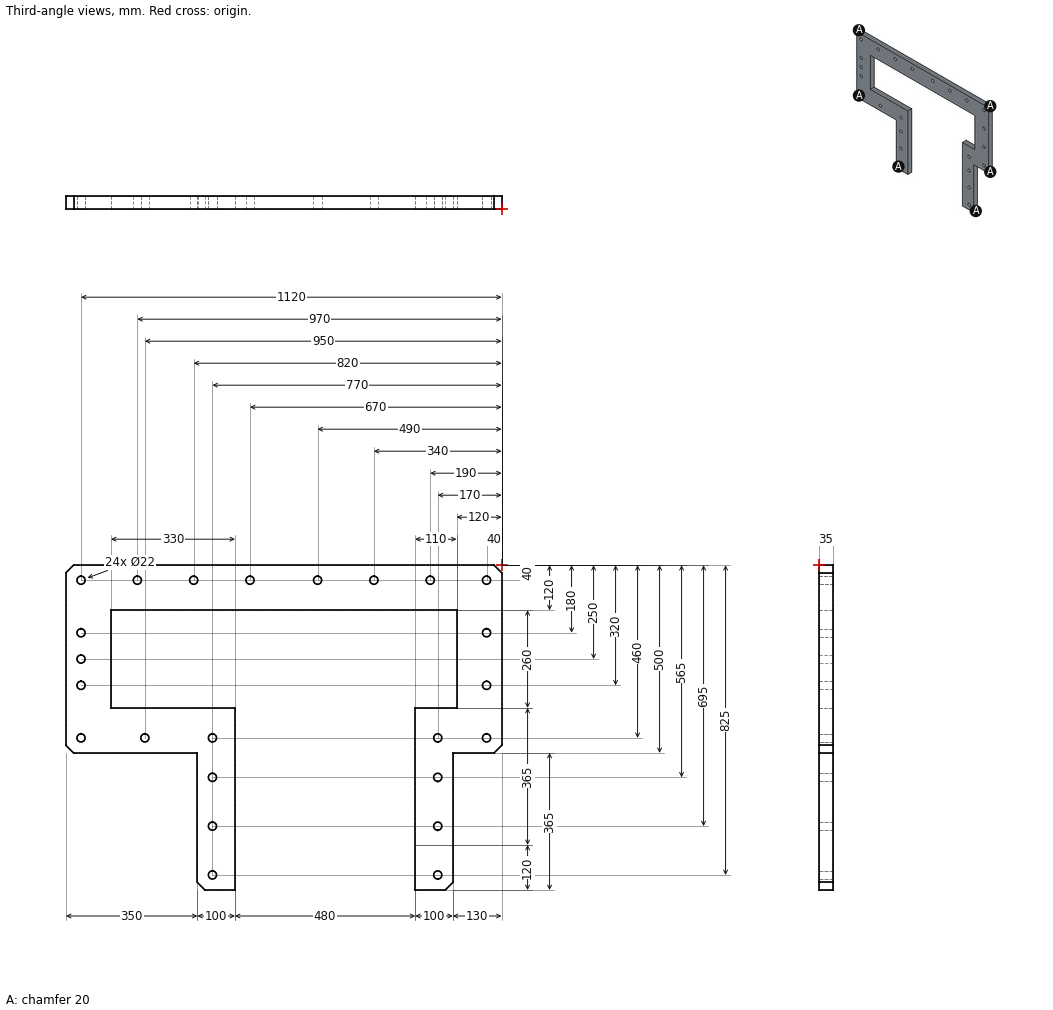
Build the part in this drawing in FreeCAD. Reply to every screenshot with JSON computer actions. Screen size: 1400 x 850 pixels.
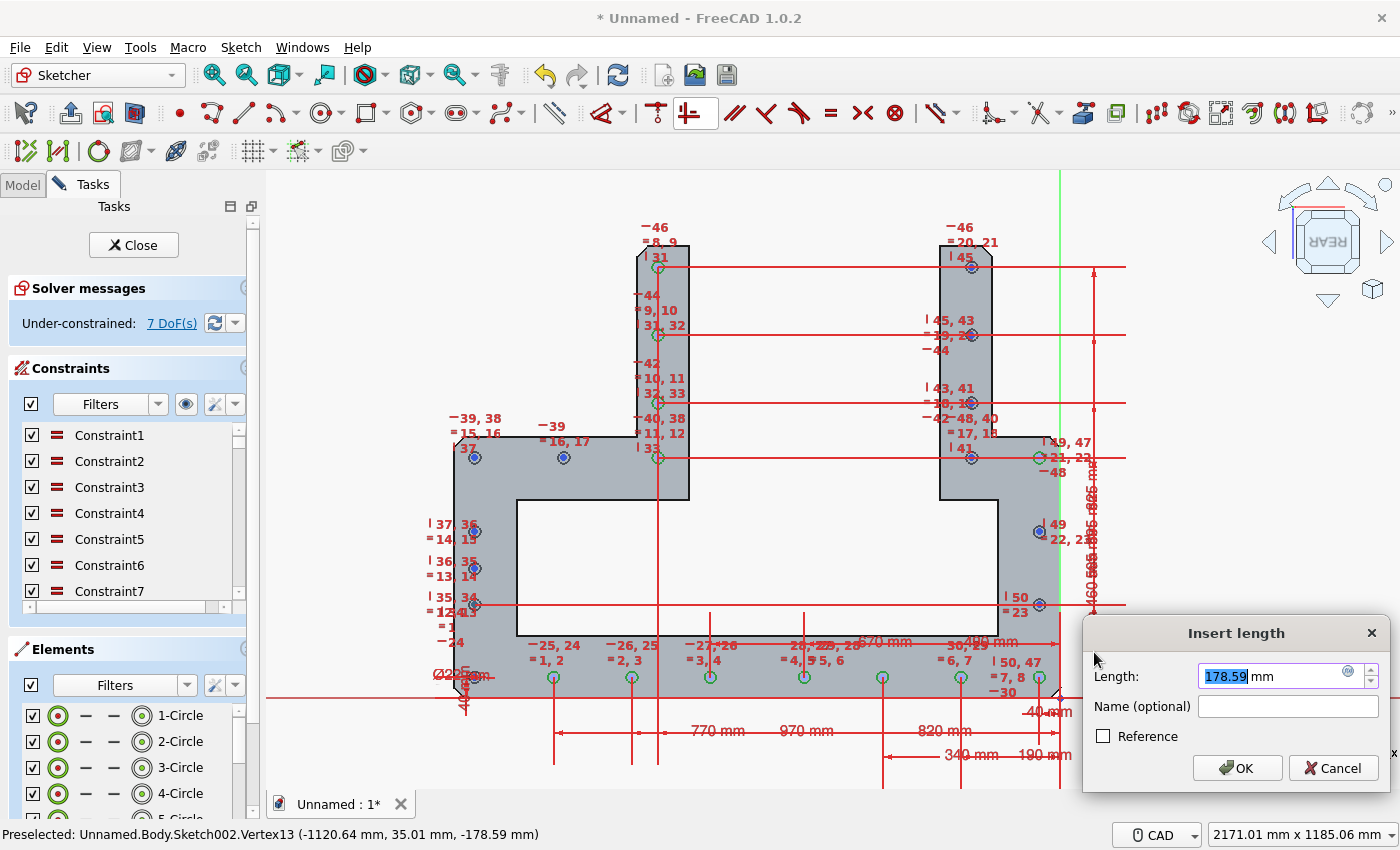
{"action": "type", "text": "180"}
{"action": "key", "text": "Return"}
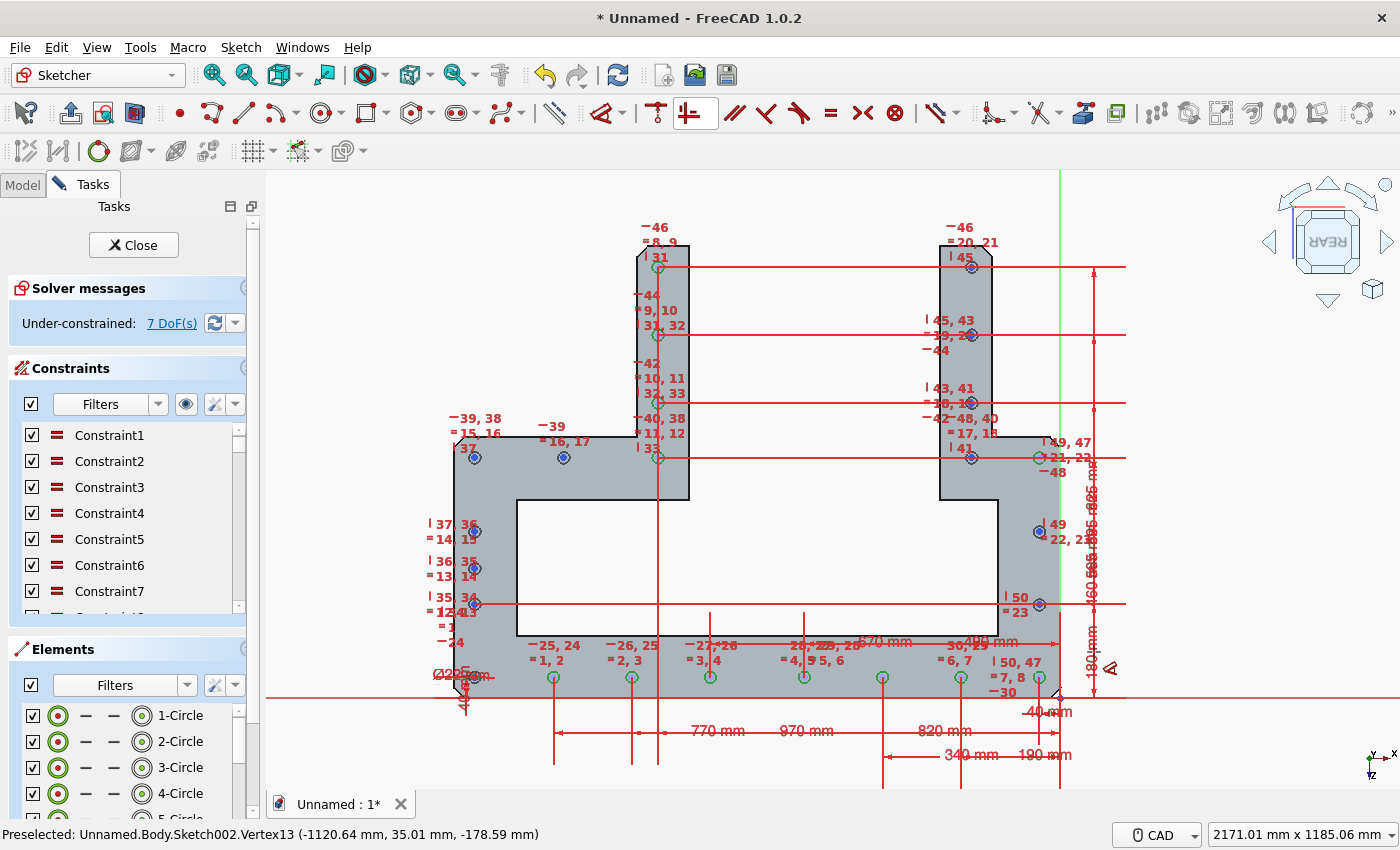
{"action": "left_click", "coordinate": [475, 569]}
{"action": "left_click", "coordinate": [1094, 604]}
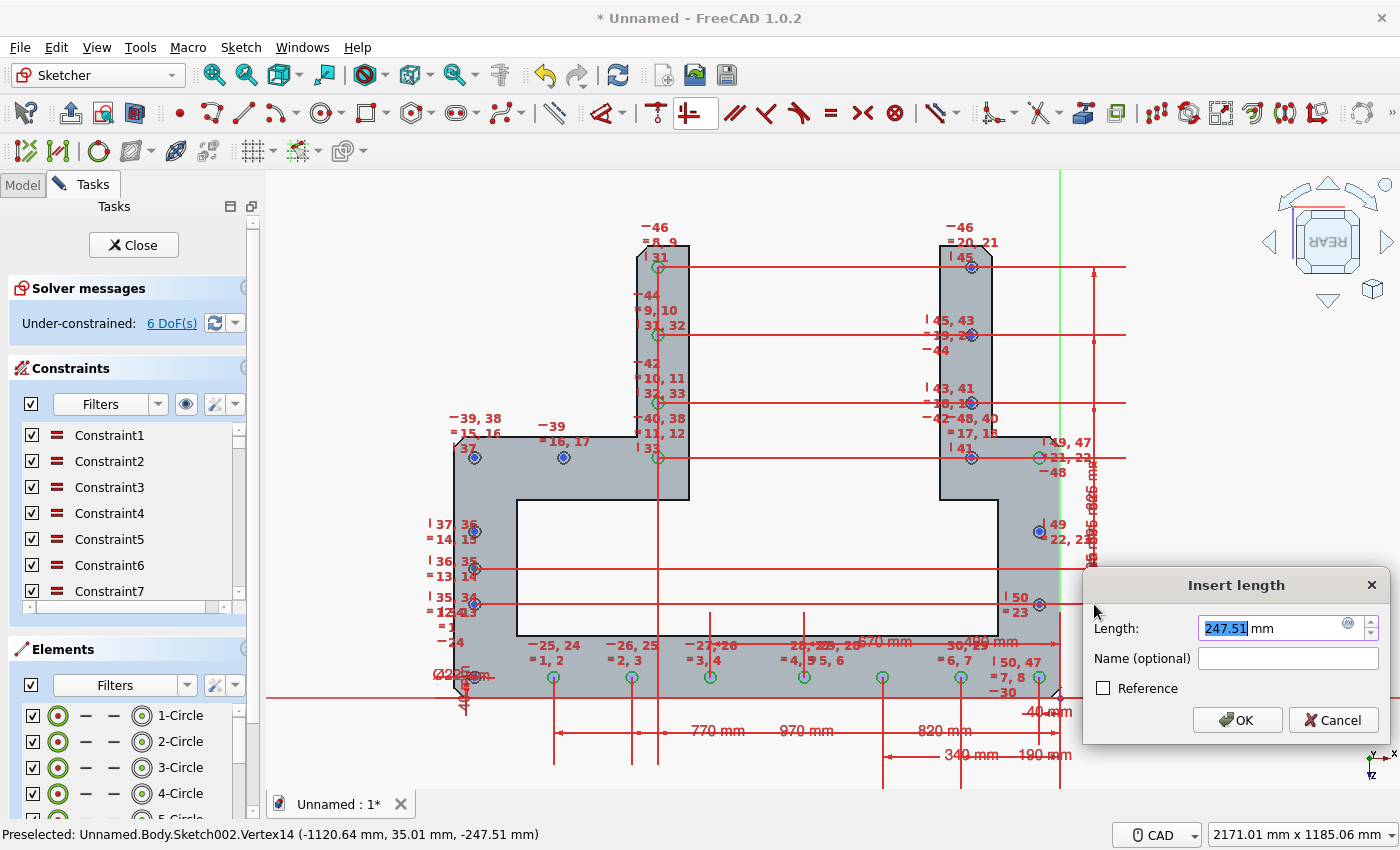
{"action": "type", "text": "250"}
{"action": "key", "text": "Return"}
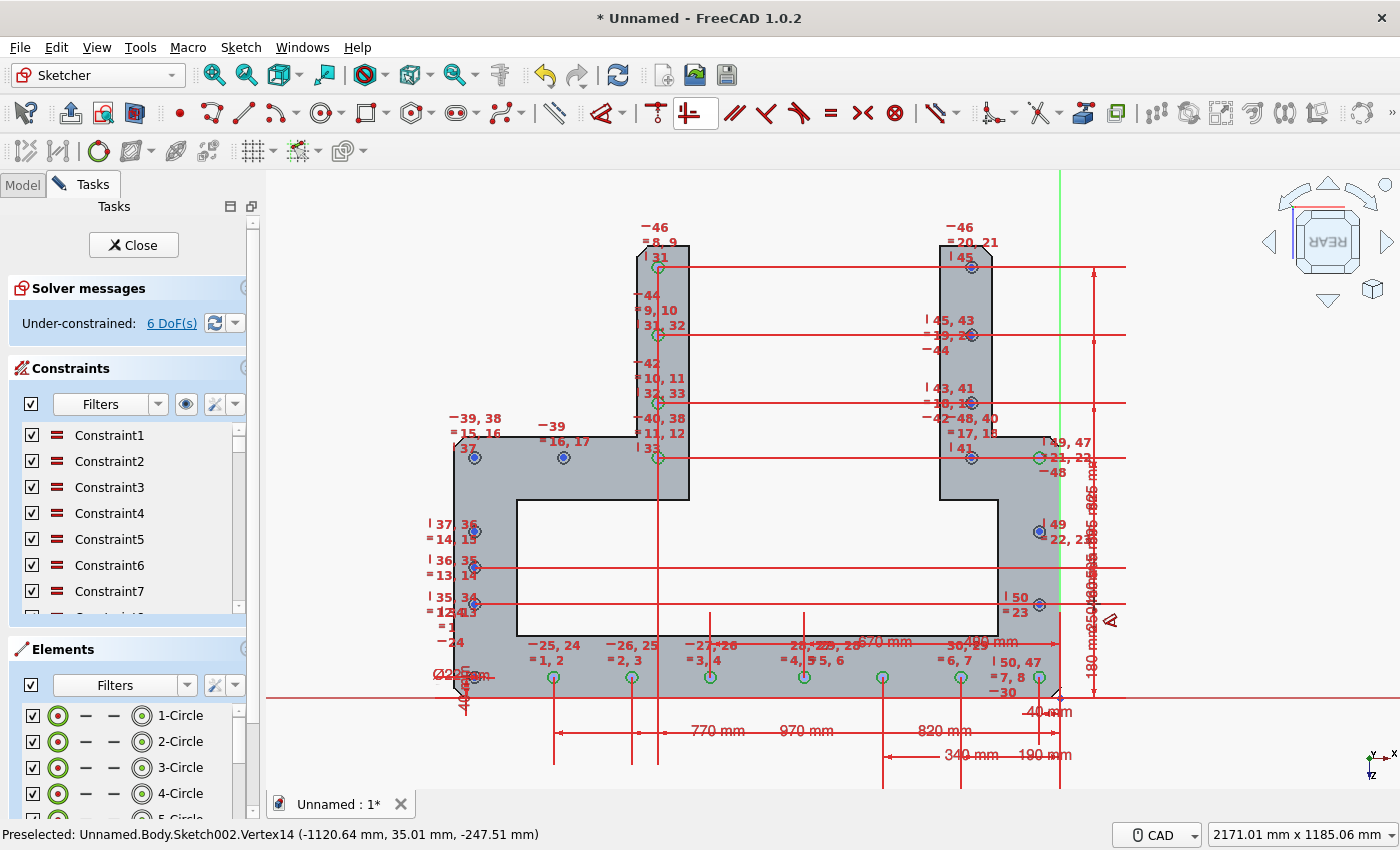
{"action": "left_click", "coordinate": [475, 532]}
{"action": "left_click", "coordinate": [1094, 673]}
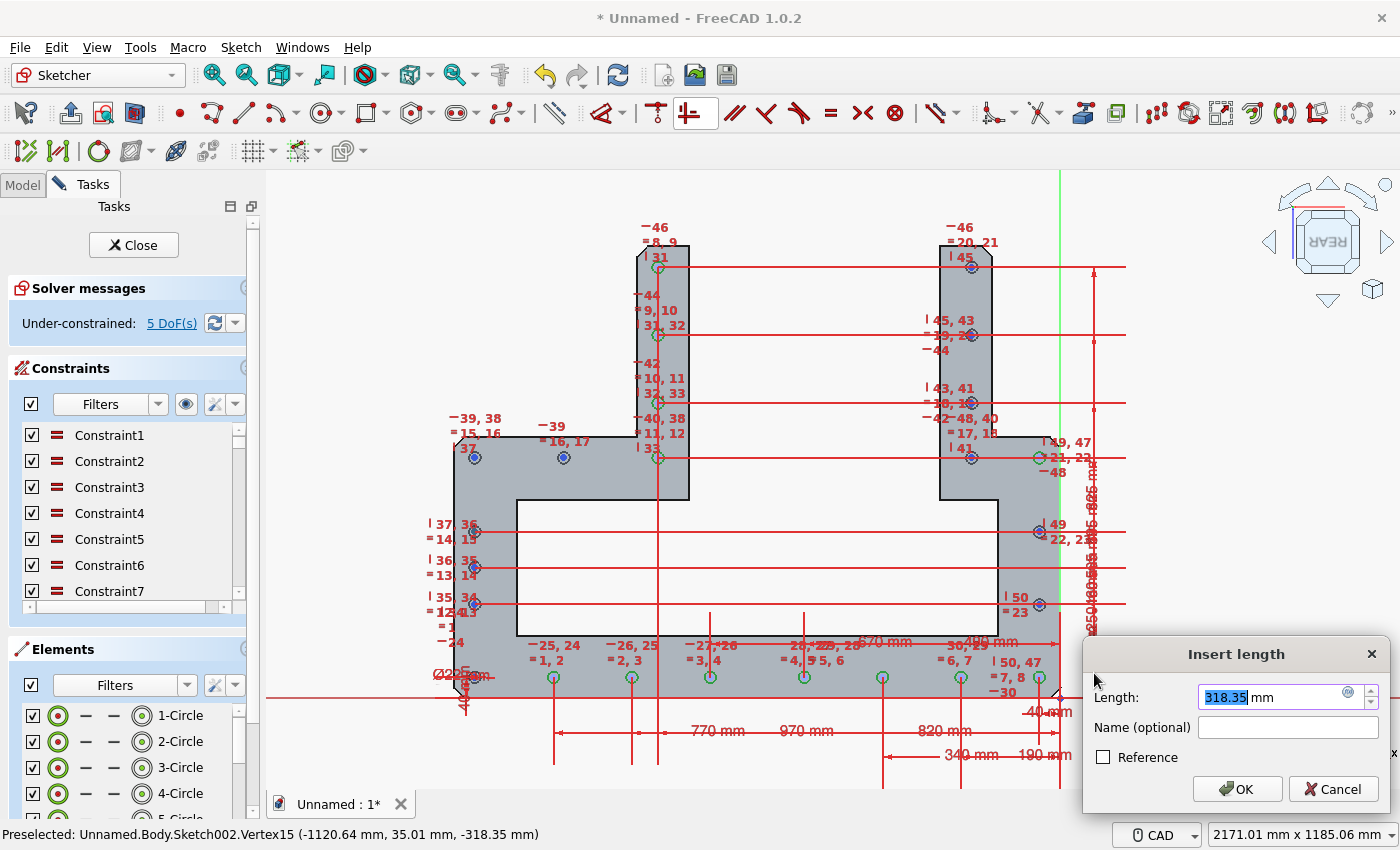
{"action": "type", "text": "320"}
{"action": "key", "text": "Return"}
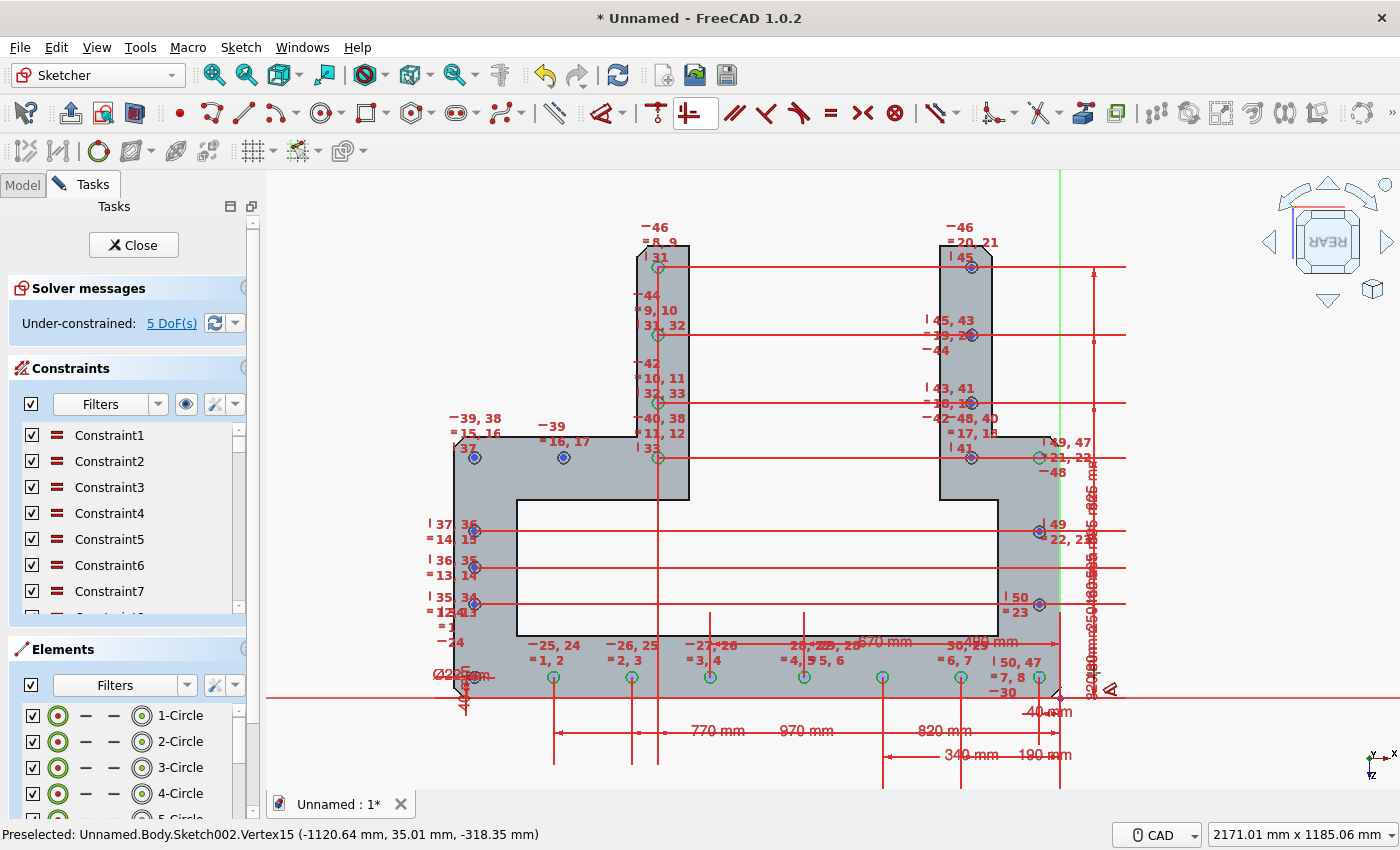
{"action": "left_click", "coordinate": [564, 458]}
{"action": "left_click", "coordinate": [638, 732]}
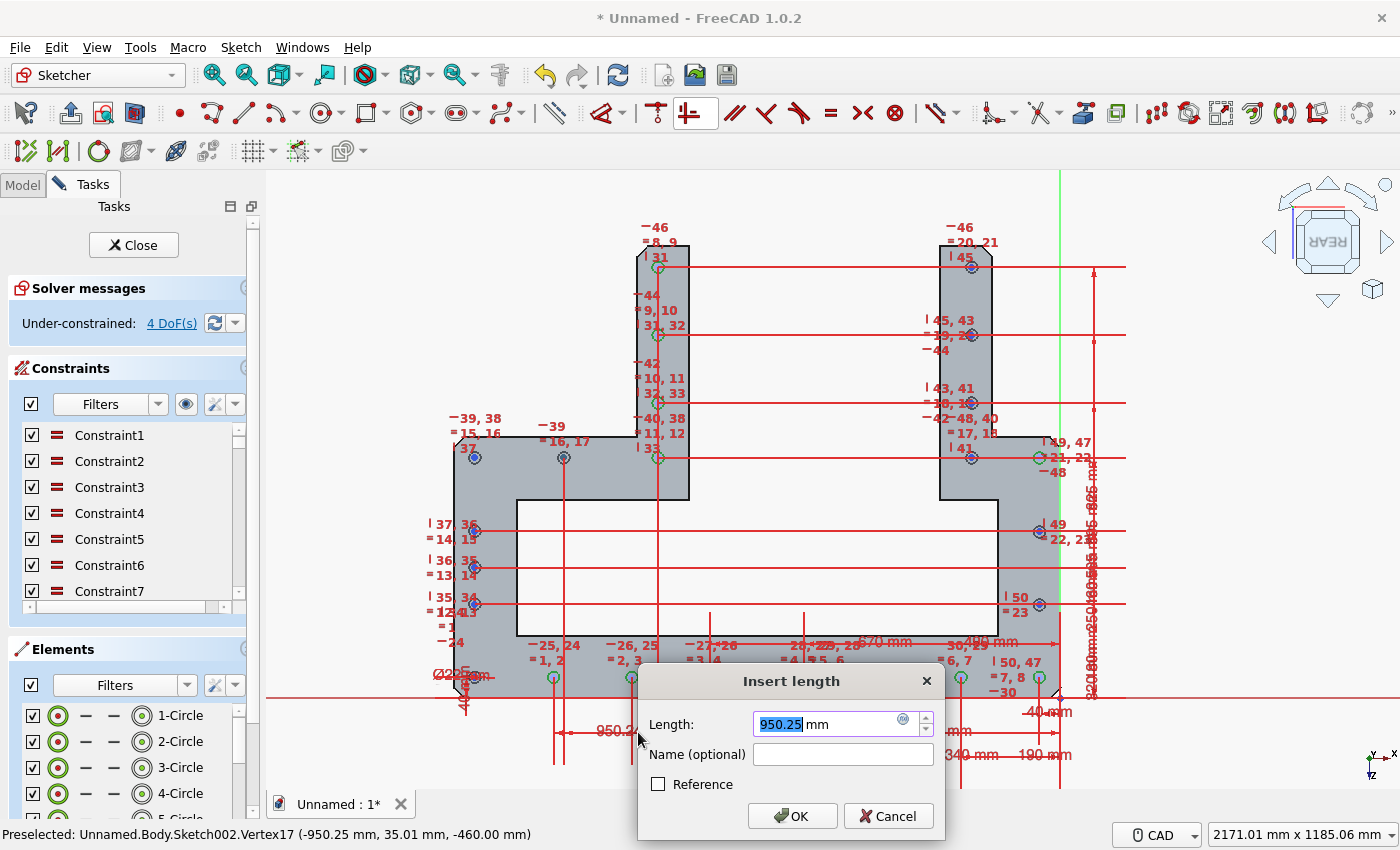
{"action": "type", "text": "950"}
{"action": "key", "text": "Return"}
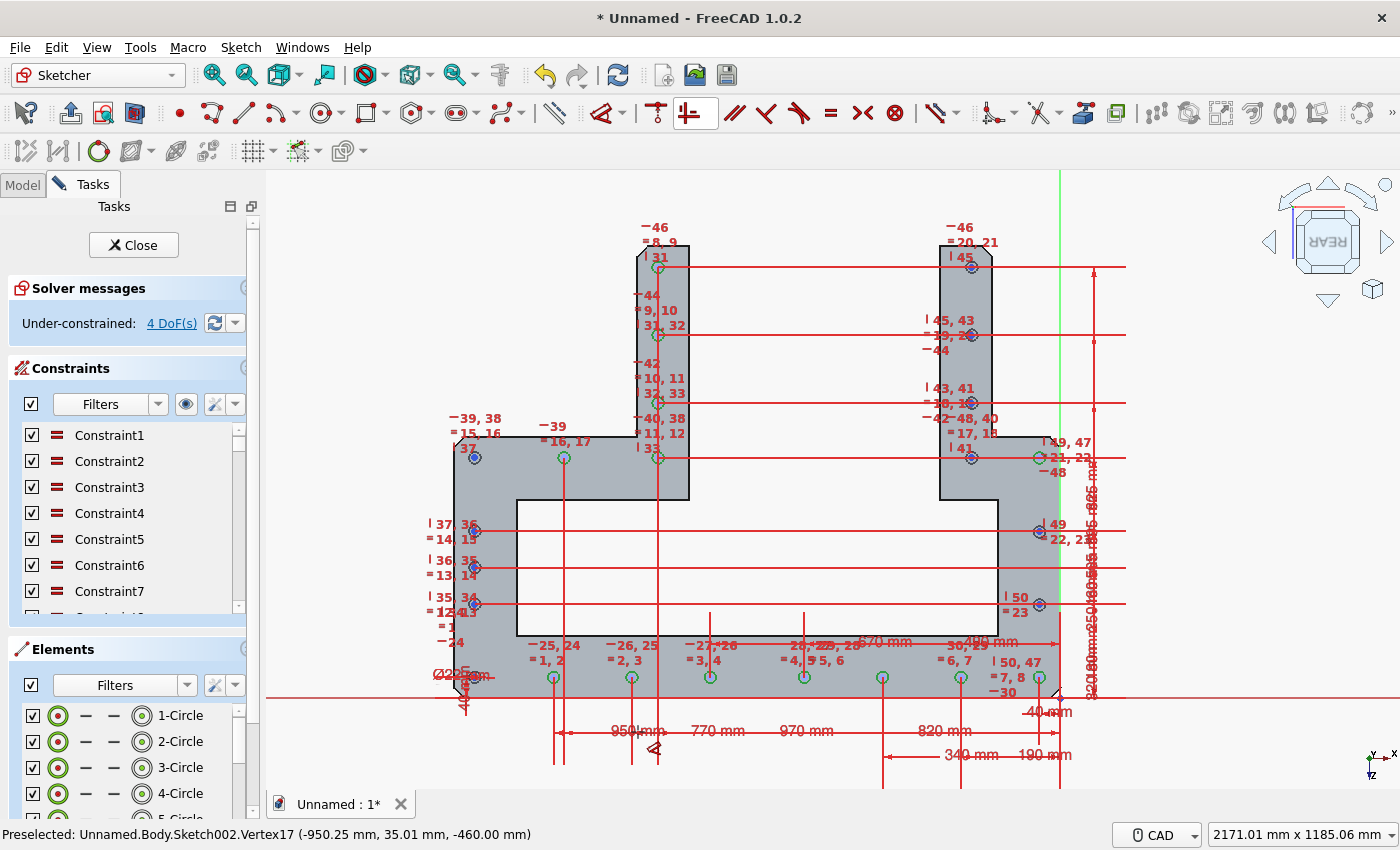
{"action": "left_click", "coordinate": [972, 458]}
{"action": "left_click", "coordinate": [1016, 424]}